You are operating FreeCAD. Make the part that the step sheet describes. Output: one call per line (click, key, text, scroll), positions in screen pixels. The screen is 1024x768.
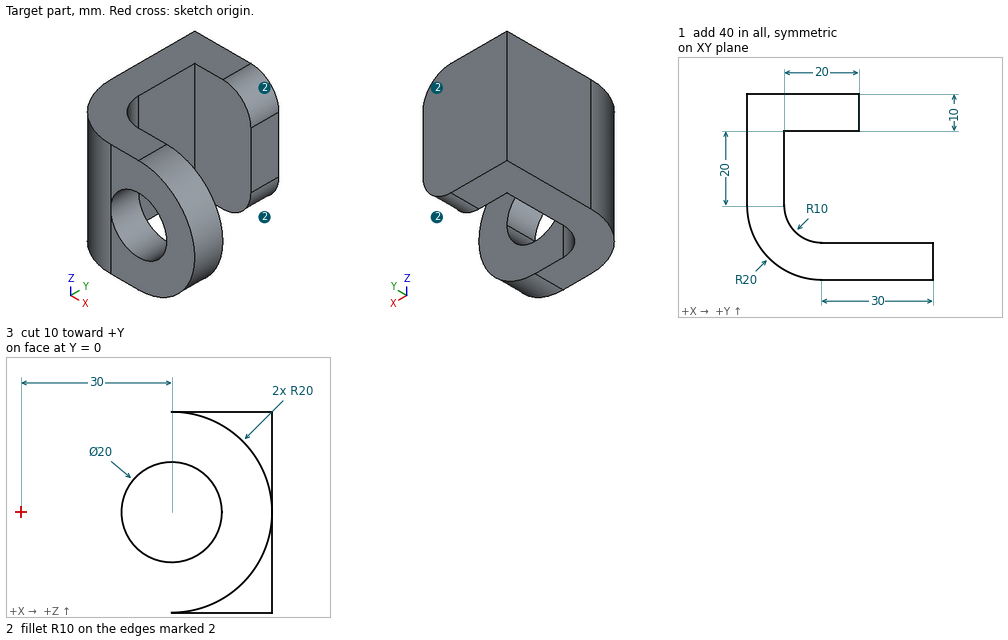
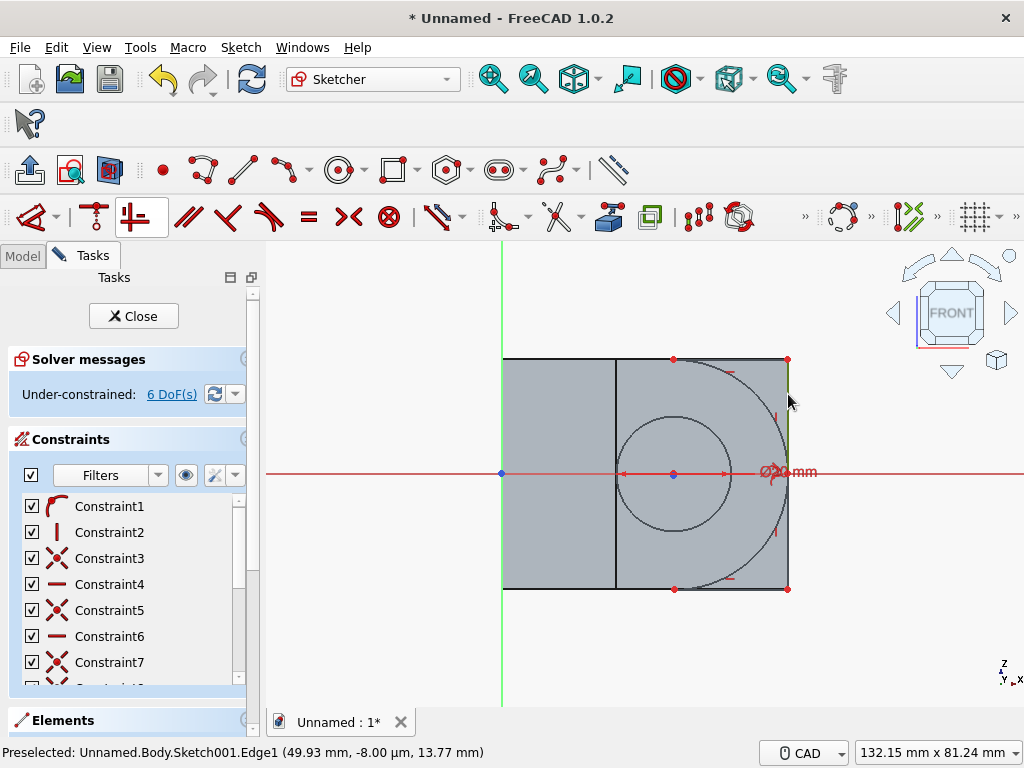
click(755, 556)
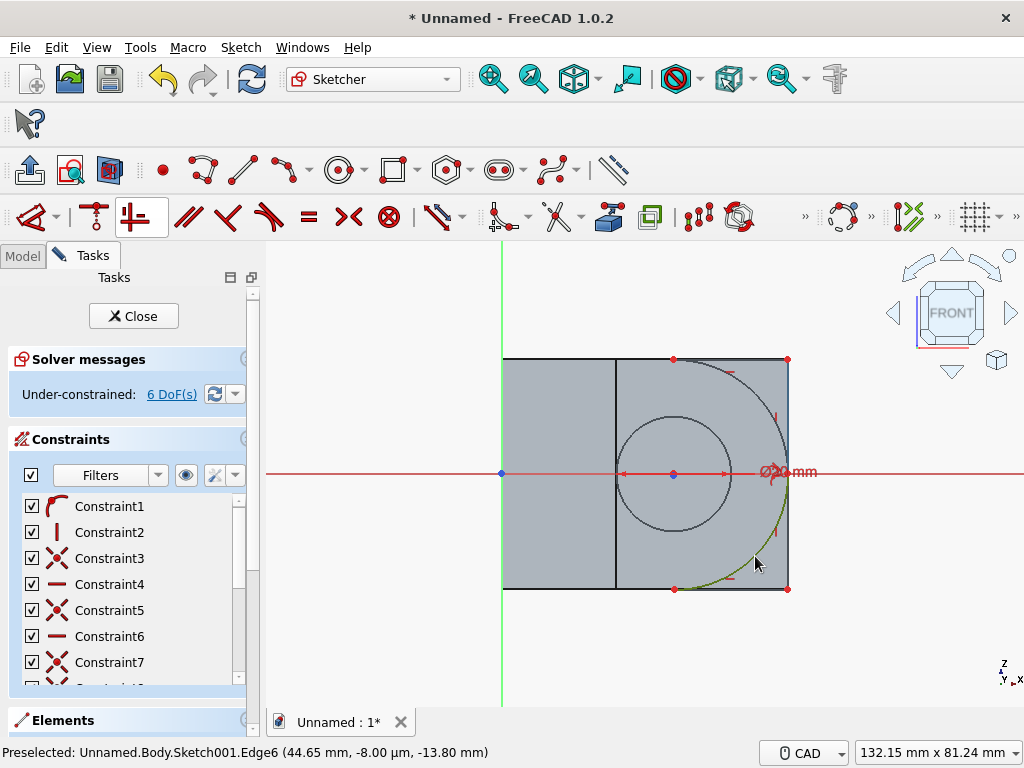
click(270, 218)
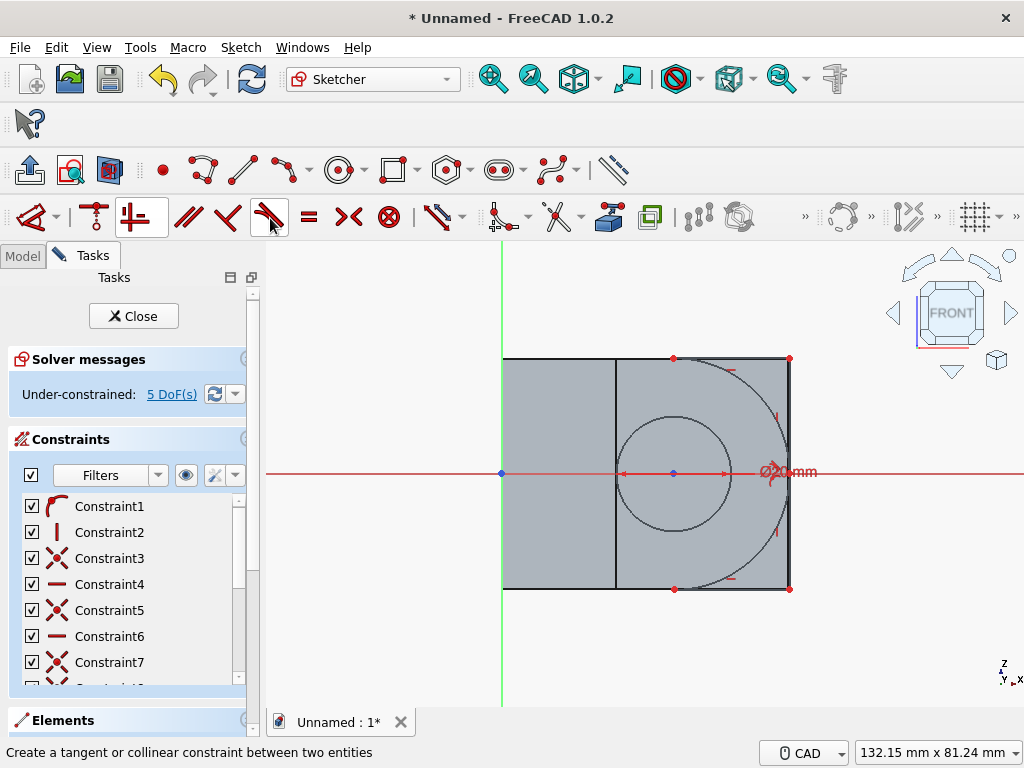
click(755, 358)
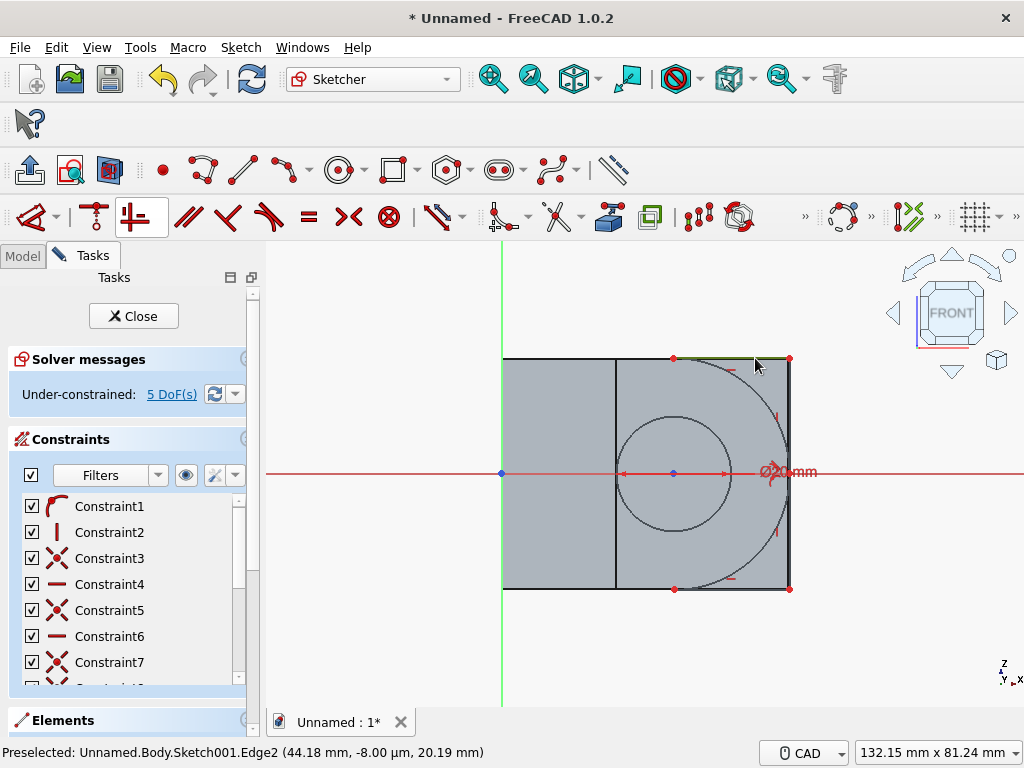
click(756, 392)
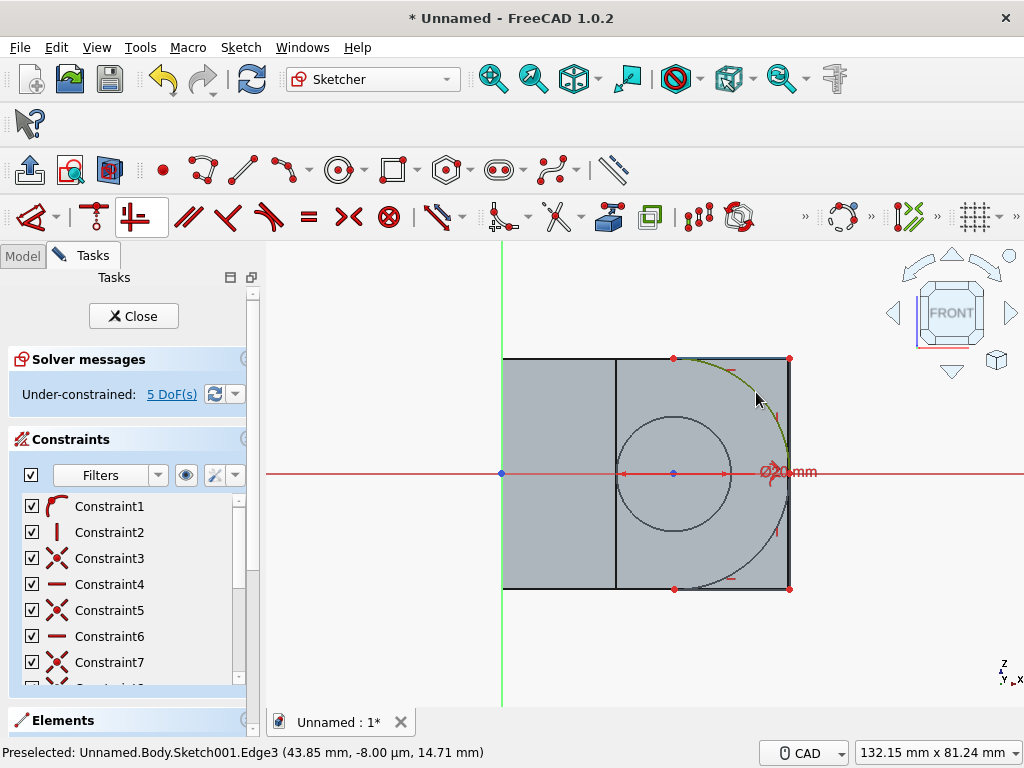
click(270, 218)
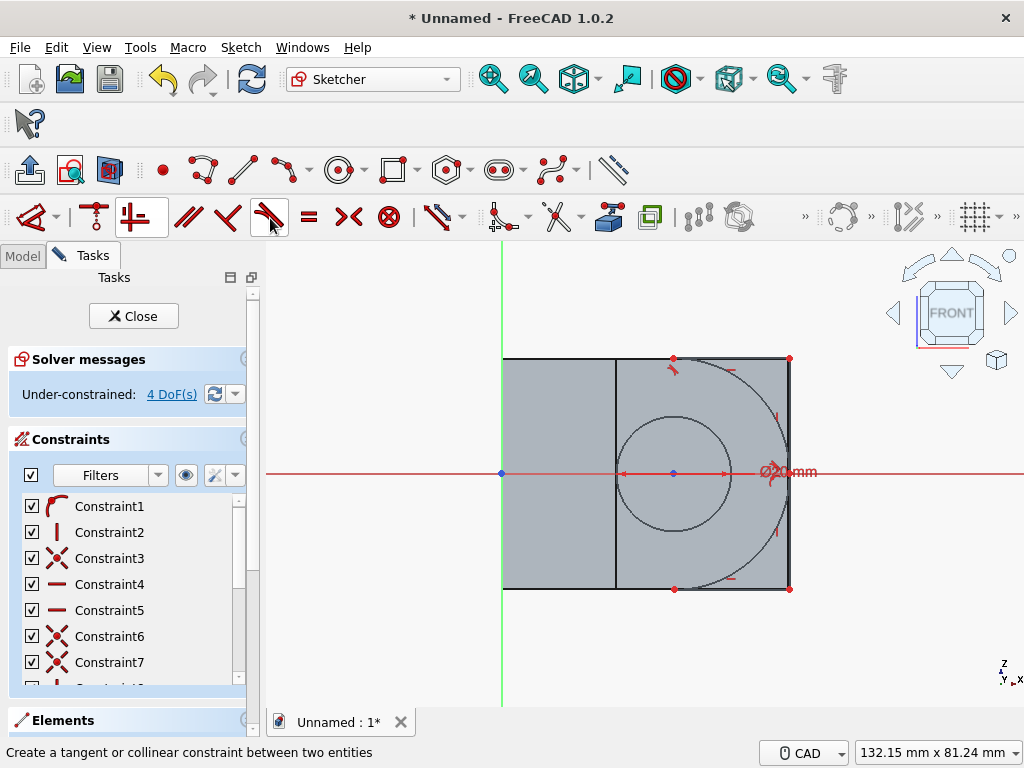
click(755, 590)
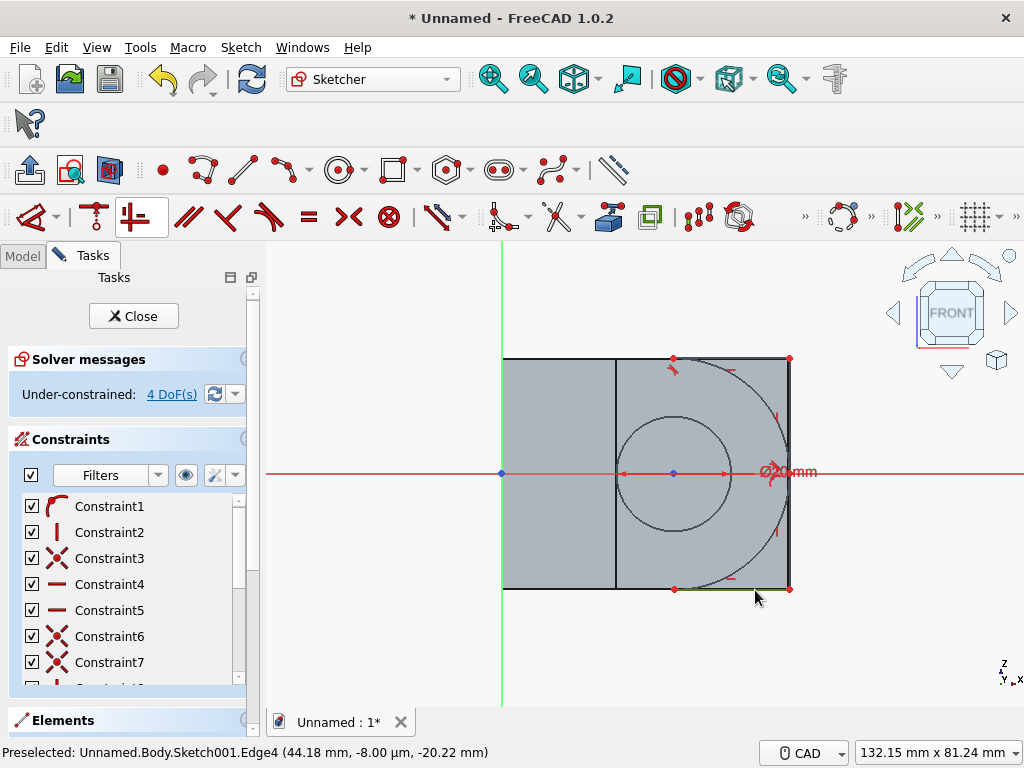
click(756, 556)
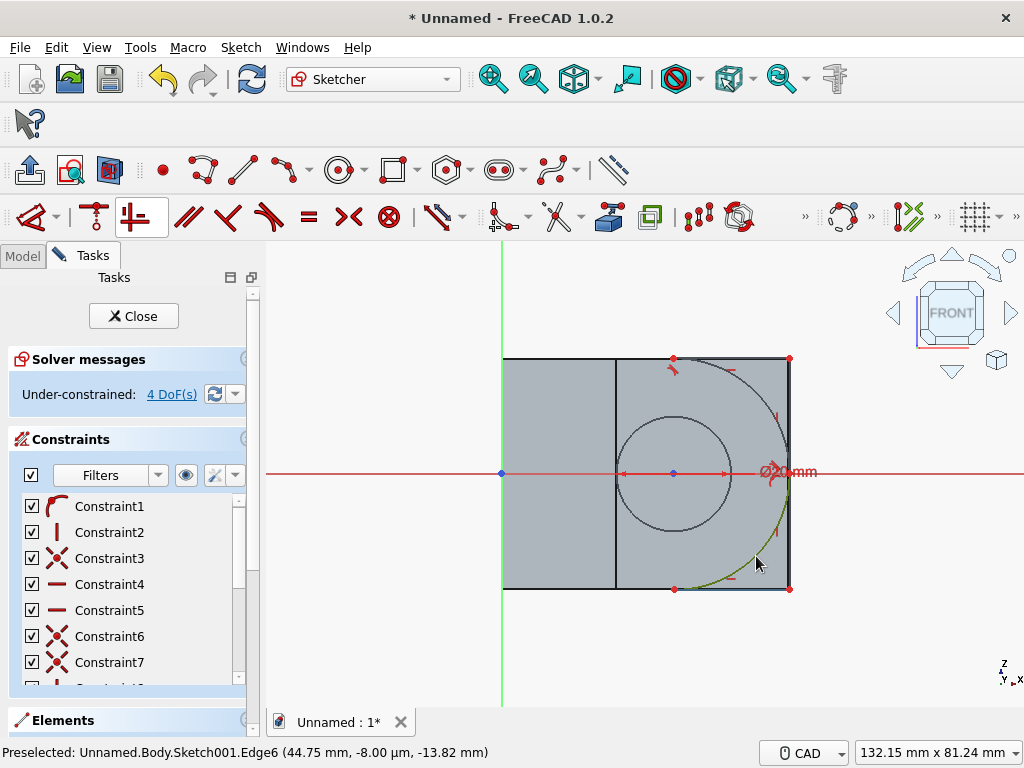
click(270, 218)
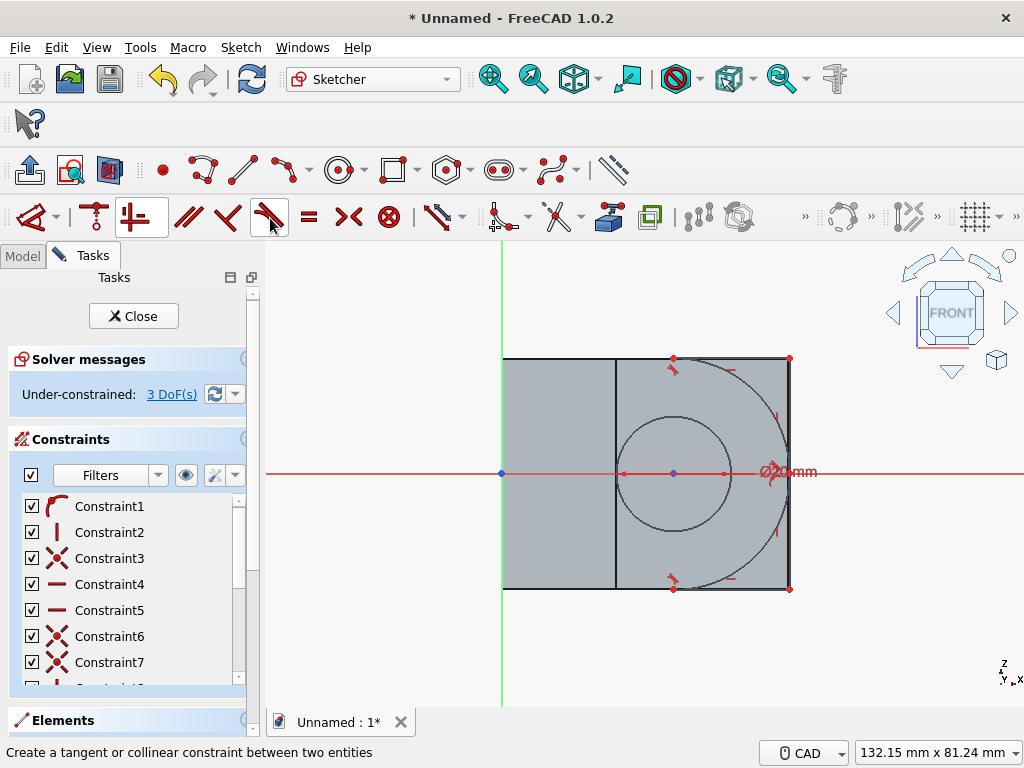
click(756, 392)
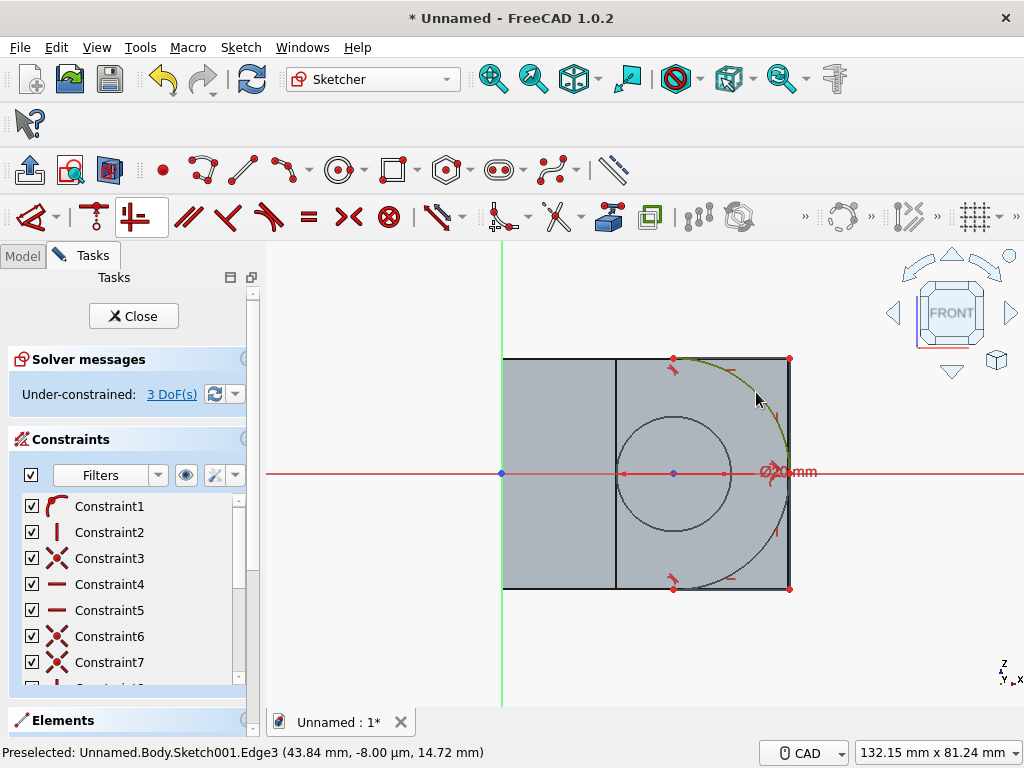
click(756, 556)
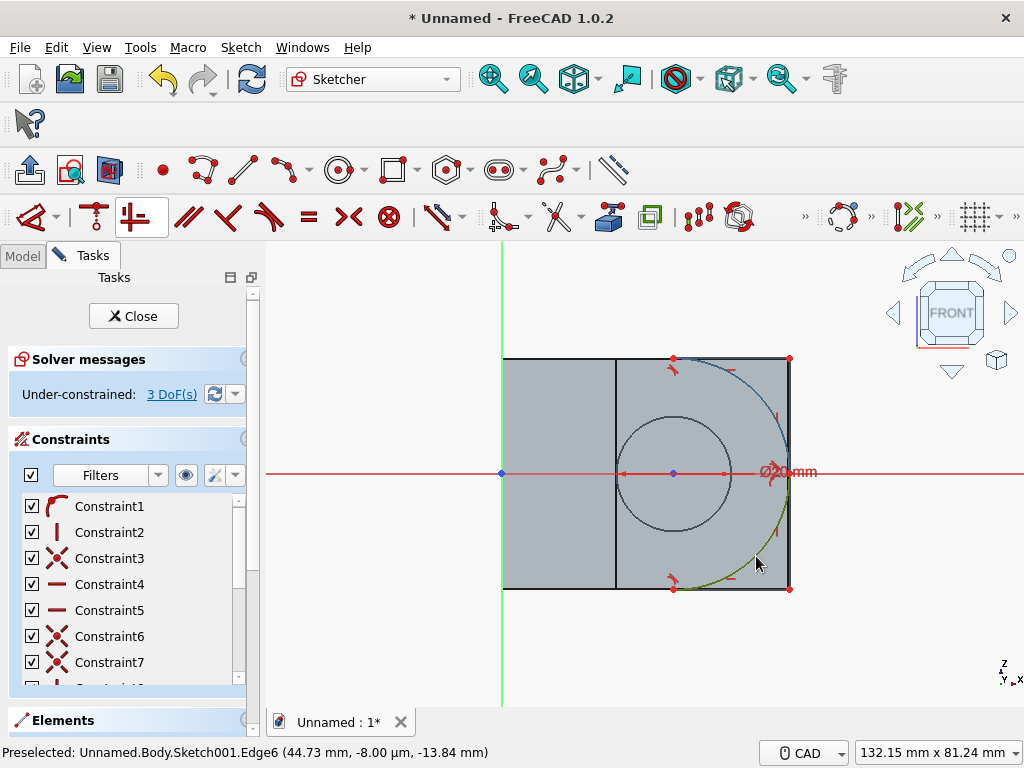
click(310, 218)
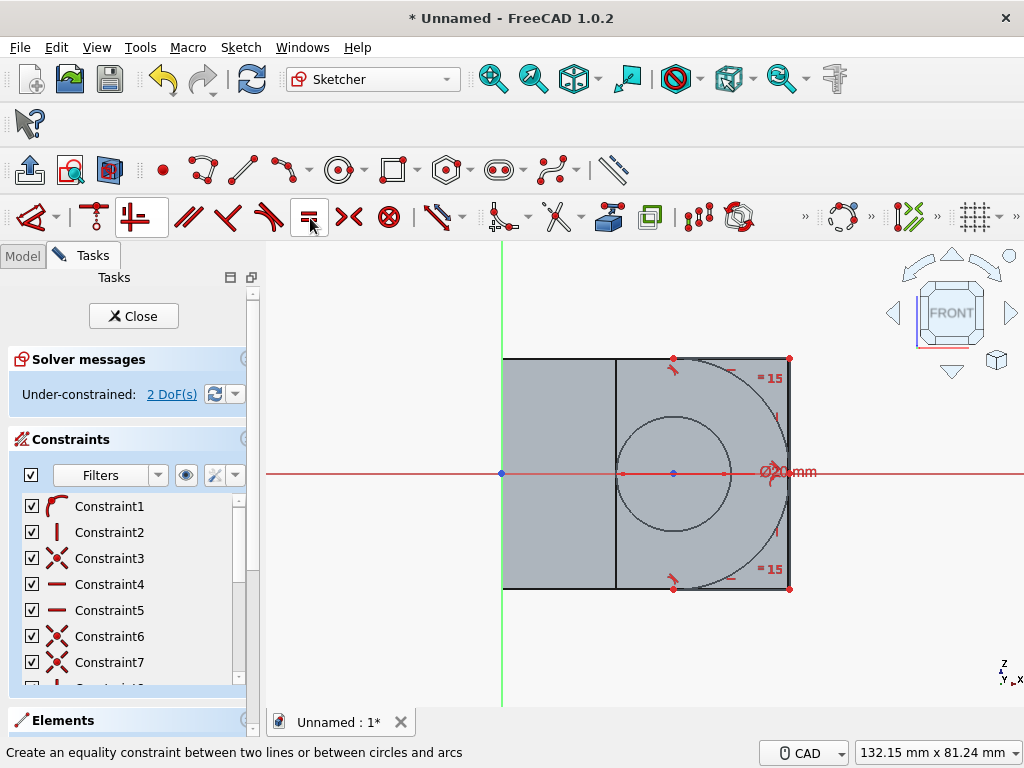
click(32, 218)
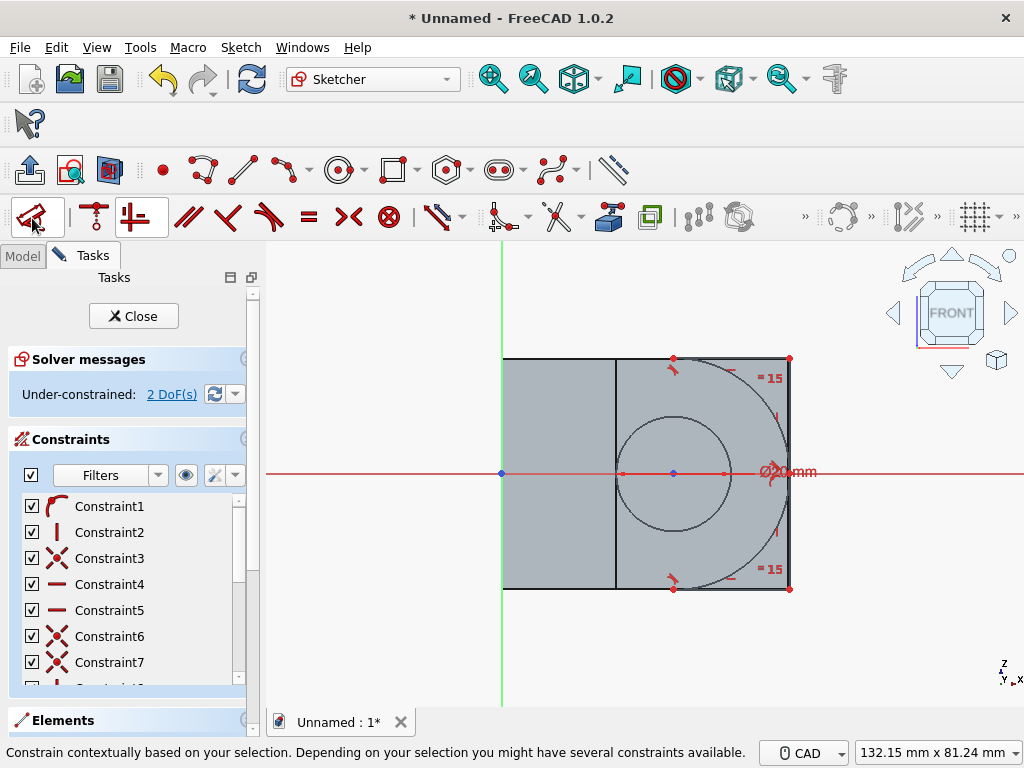
click(777, 421)
click(805, 406)